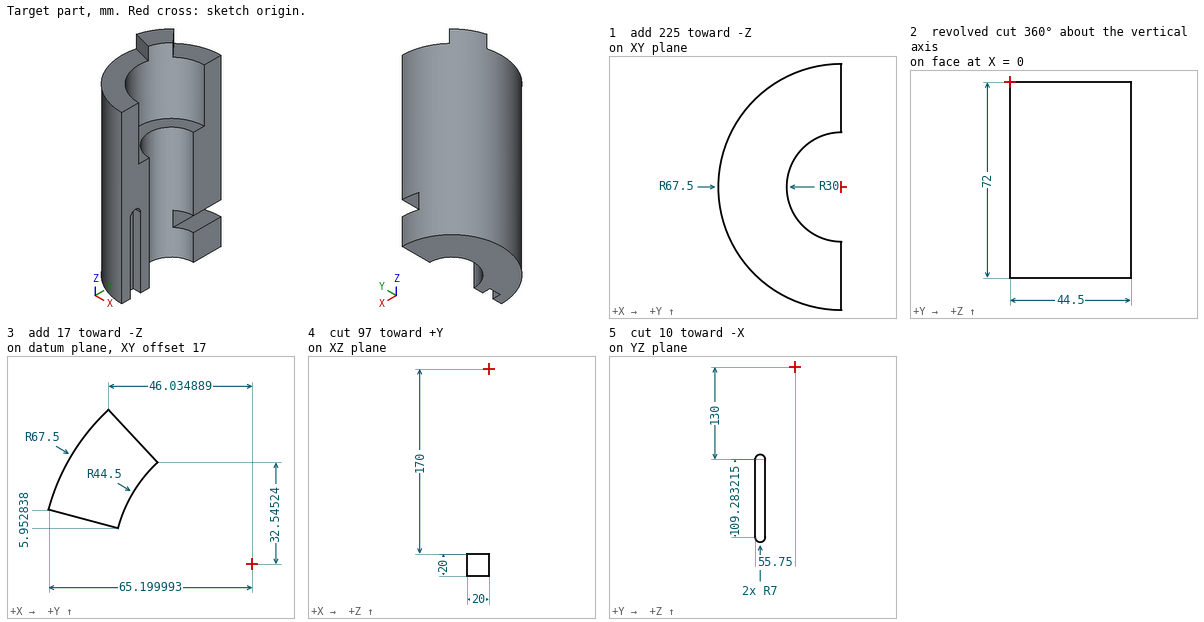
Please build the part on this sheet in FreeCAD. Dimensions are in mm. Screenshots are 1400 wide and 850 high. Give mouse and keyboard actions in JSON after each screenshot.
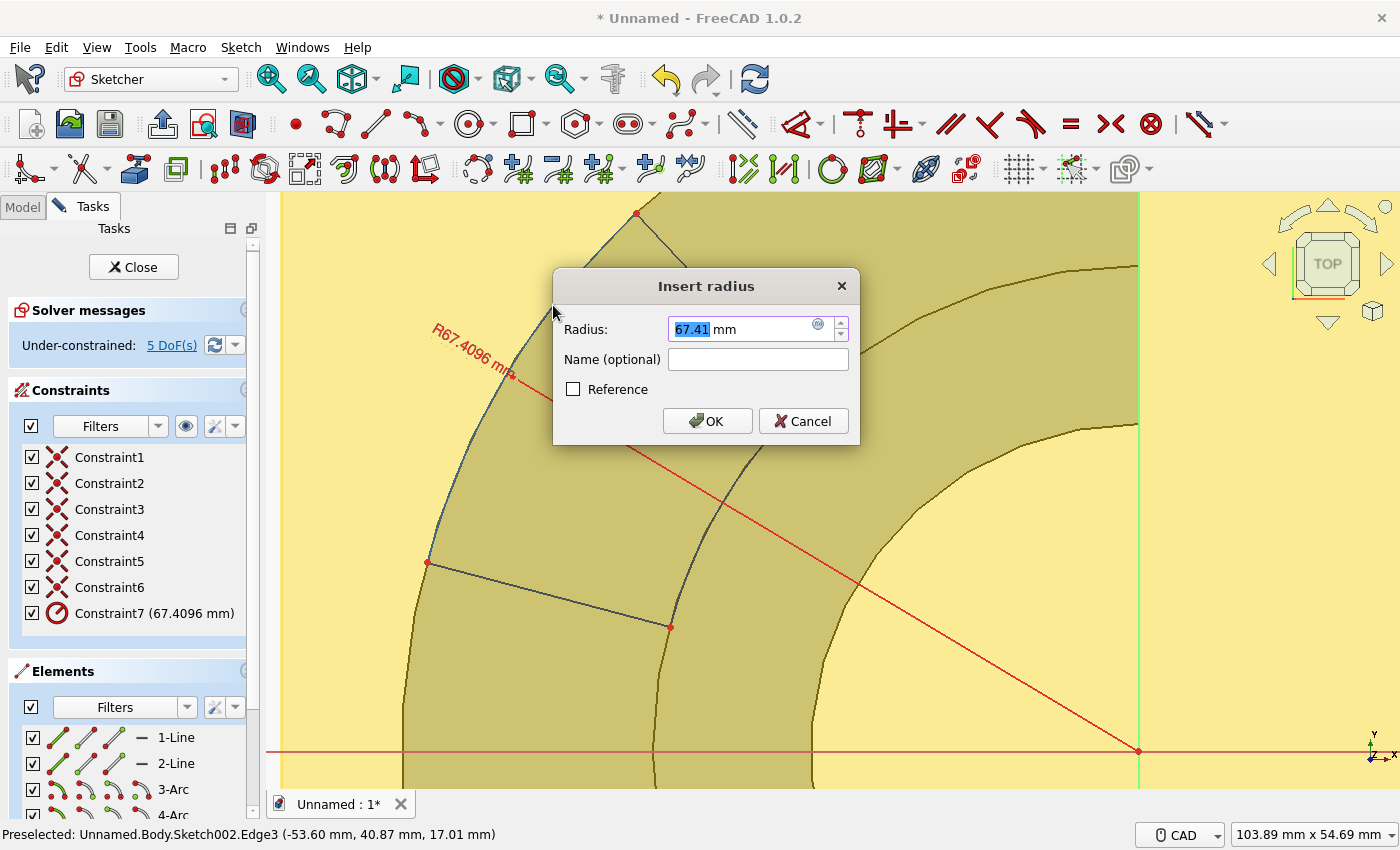
{"action": "type", "text": "67.5"}
{"action": "key", "text": "Return"}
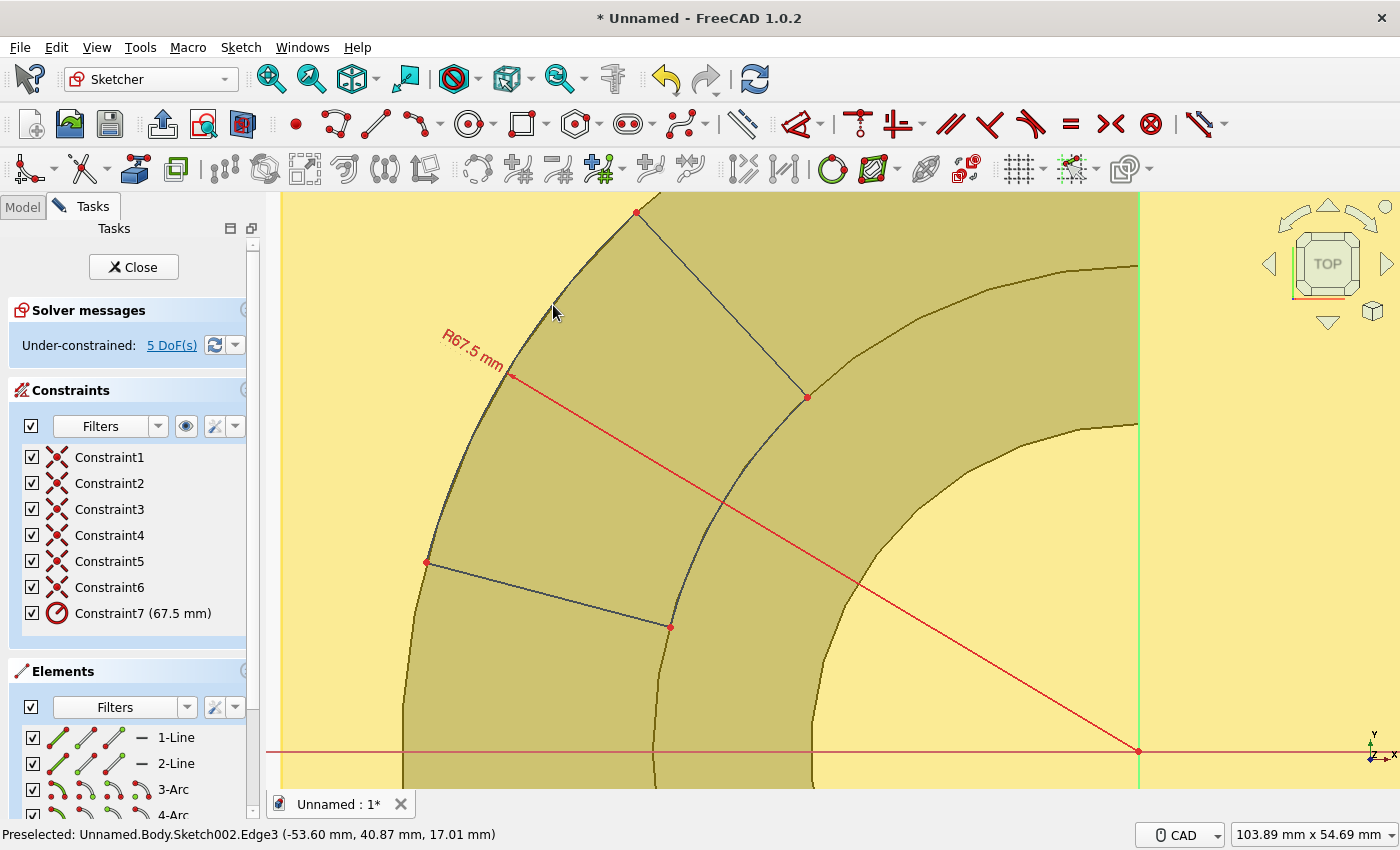
{"action": "left_click", "coordinate": [753, 458]}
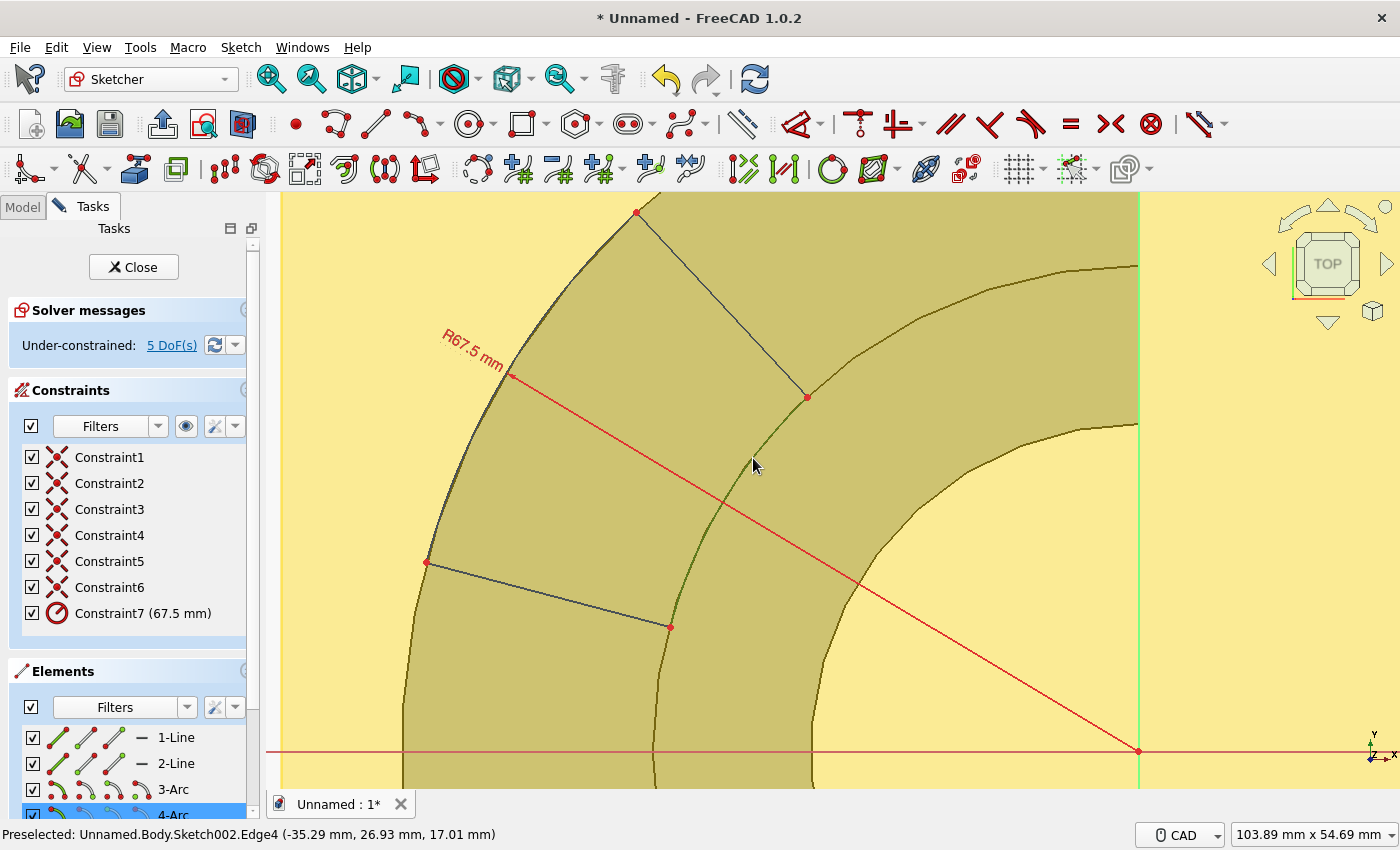
{"action": "key", "text": "k r"}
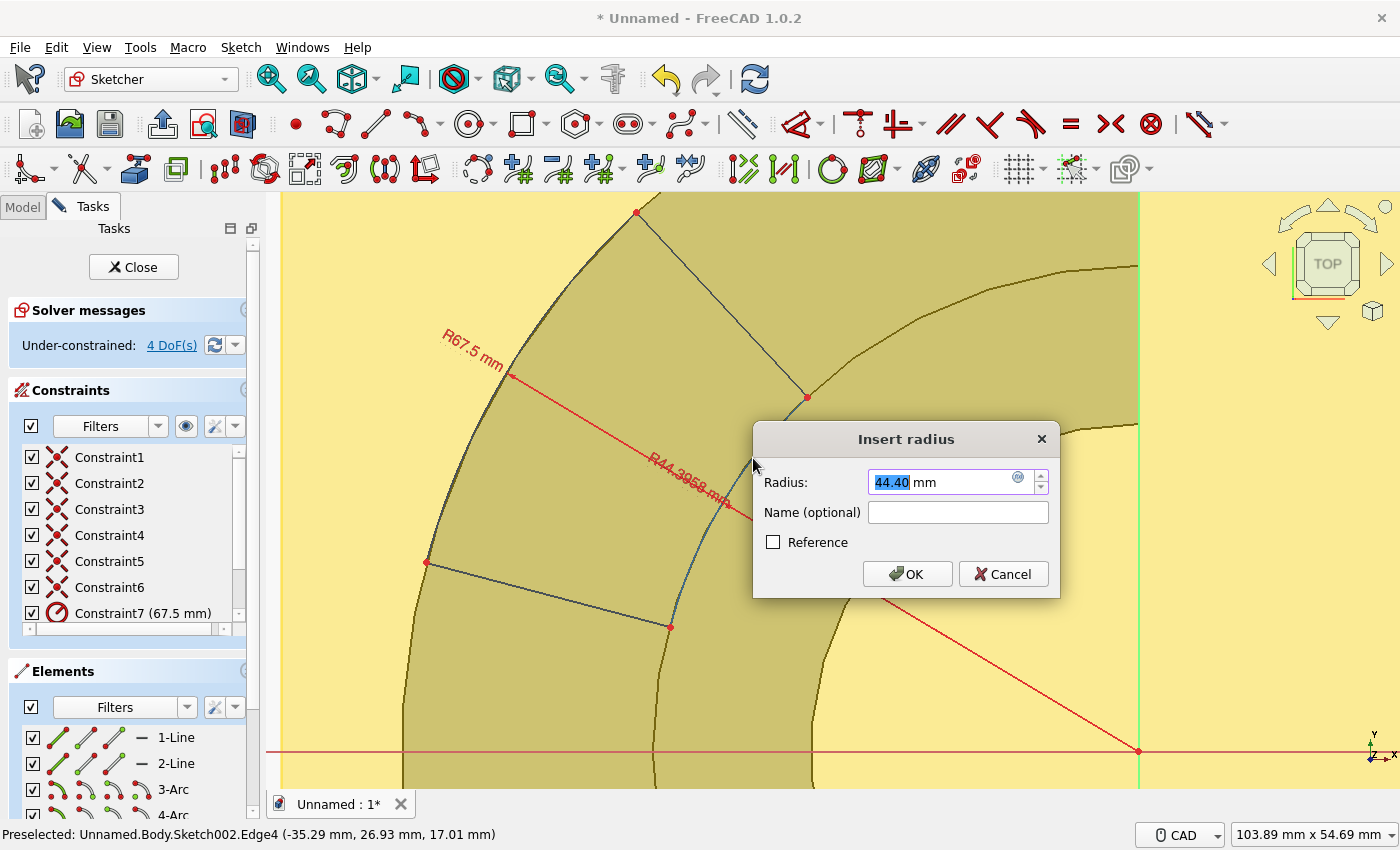
{"action": "type", "text": "44.5"}
{"action": "key", "text": "Return"}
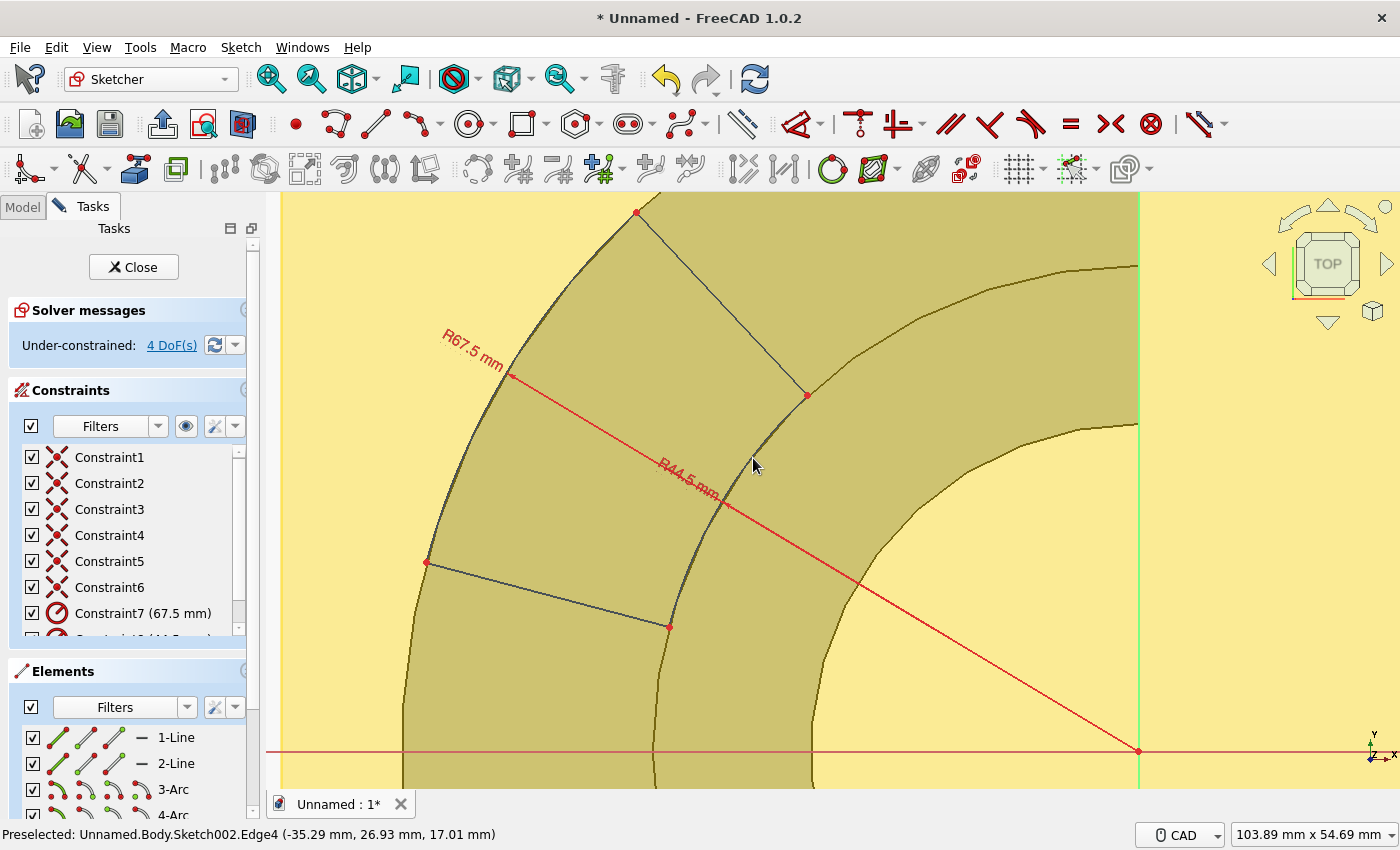
{"action": "left_click", "coordinate": [808, 396]}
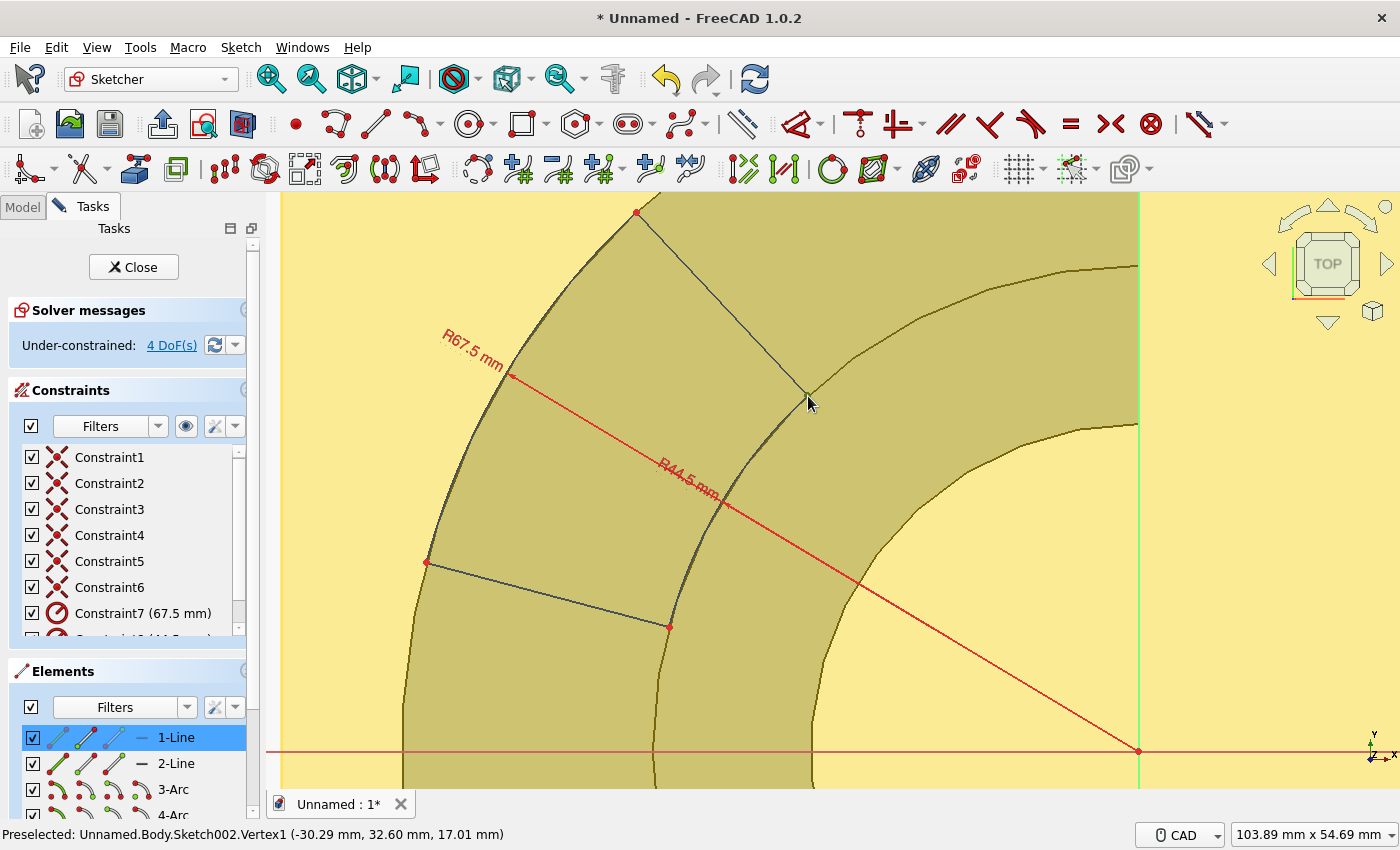
{"action": "key", "text": "i"}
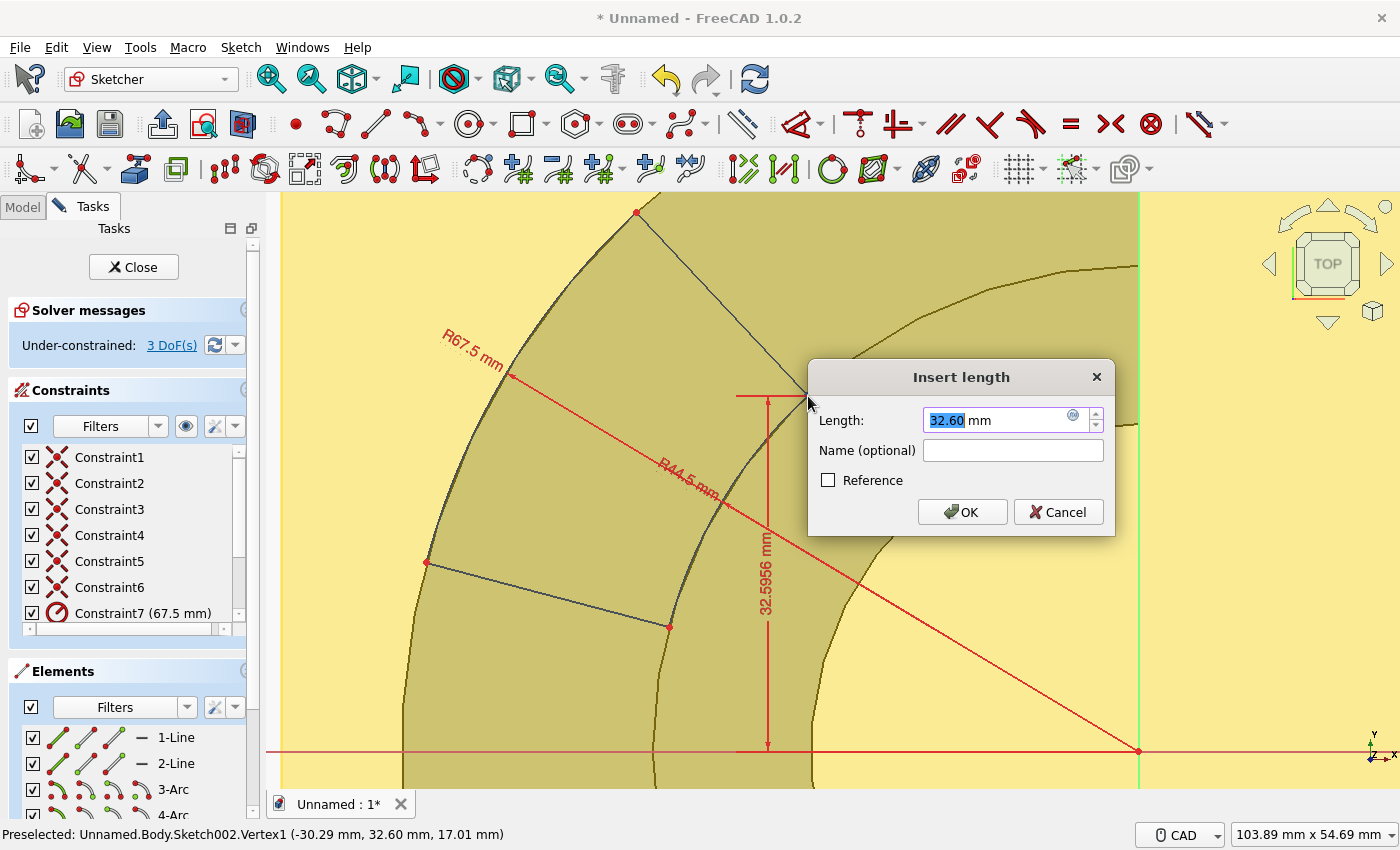
{"action": "type", "text": "32.54524"}
{"action": "key", "text": "Return"}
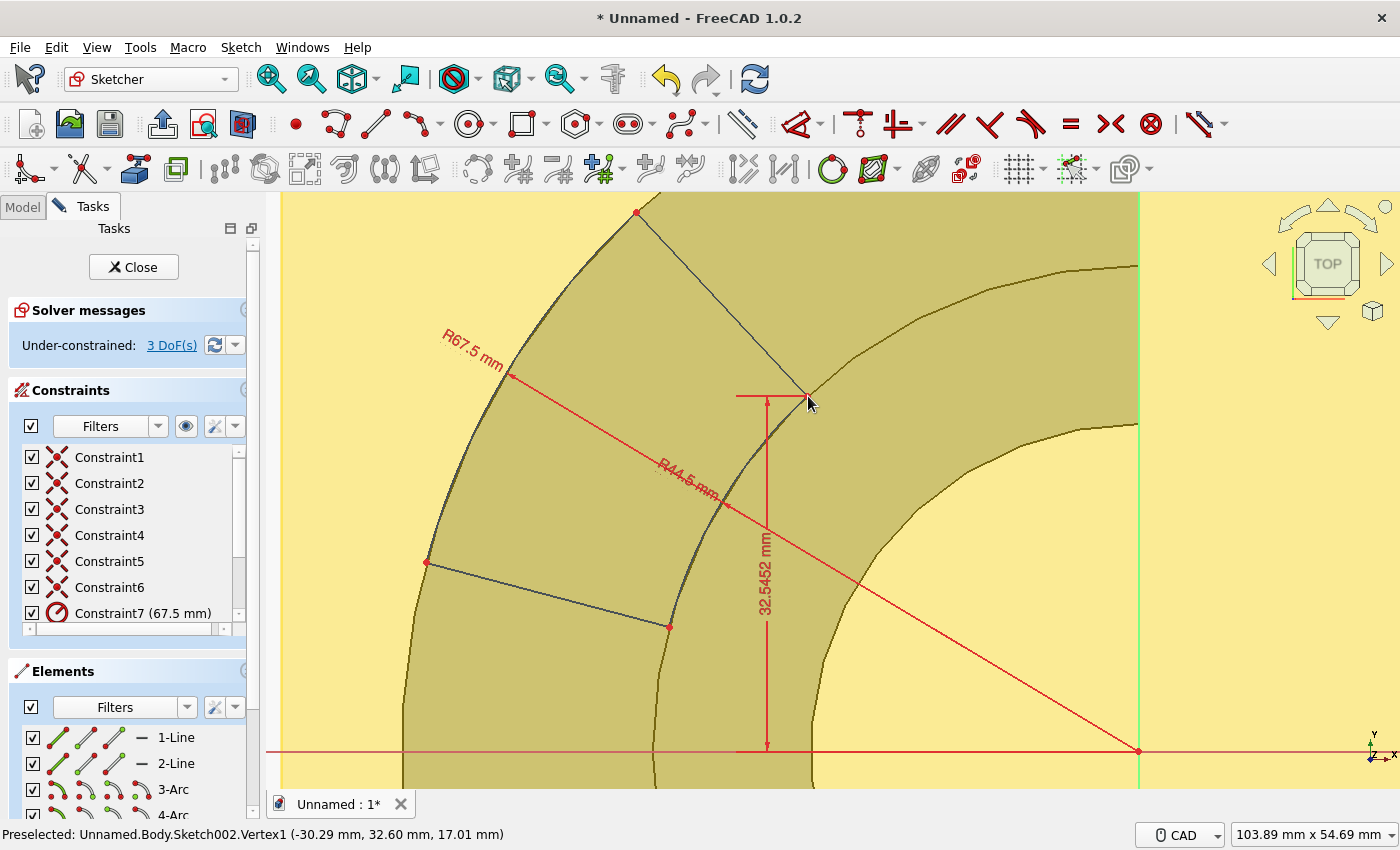
{"action": "left_click", "coordinate": [499, 582]}